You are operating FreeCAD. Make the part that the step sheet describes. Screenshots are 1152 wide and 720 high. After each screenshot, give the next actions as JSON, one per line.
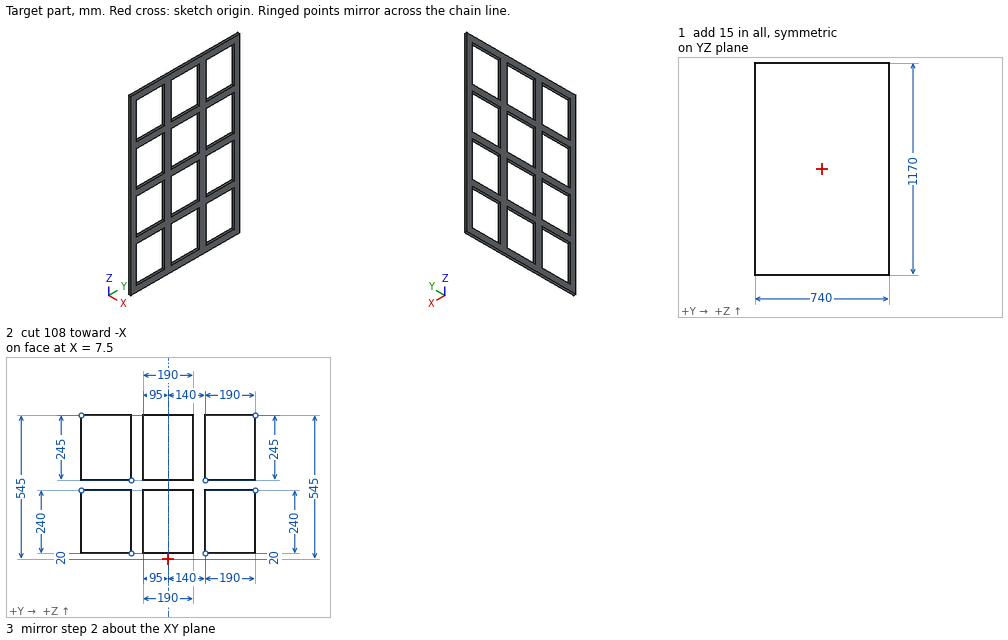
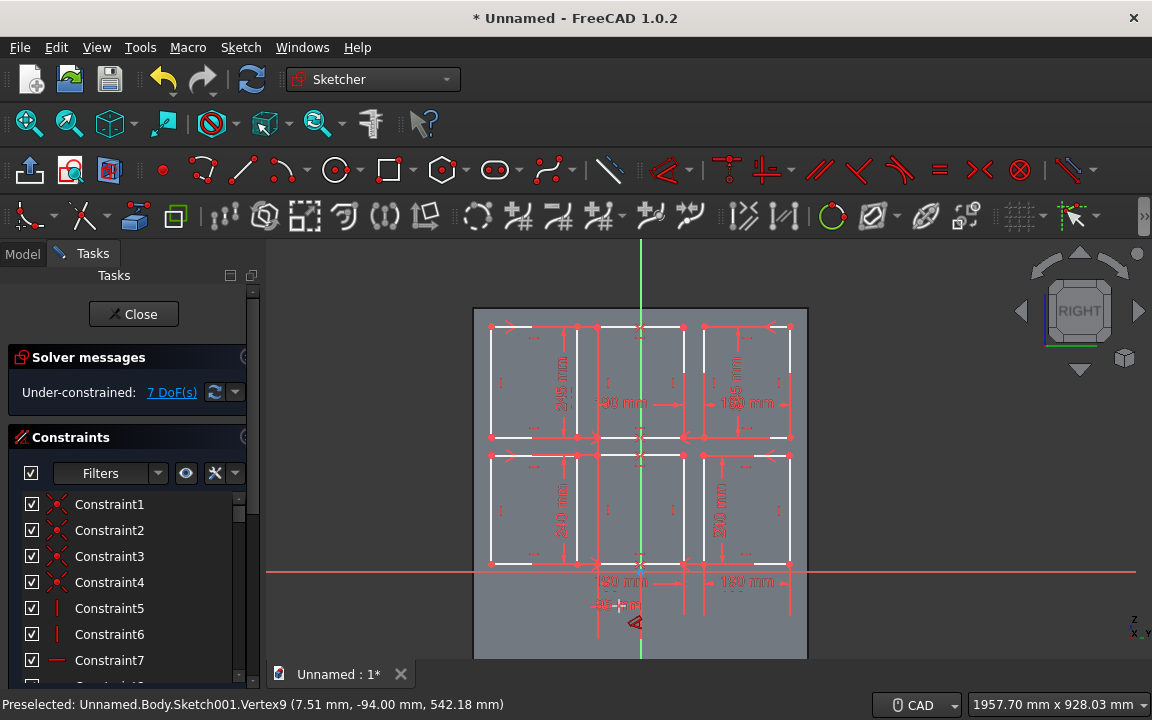
{"action": "left_click", "coordinate": [598, 455]}
{"action": "left_click", "coordinate": [619, 630]}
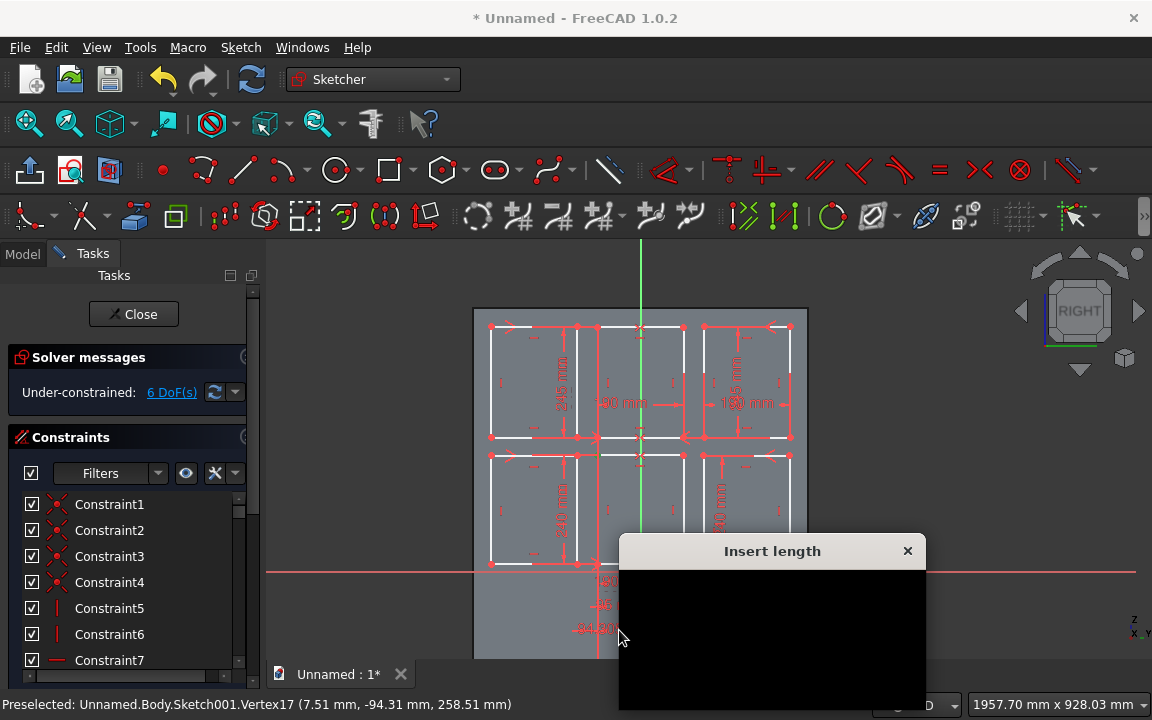
{"action": "type", "text": "95"}
{"action": "key", "text": "Return"}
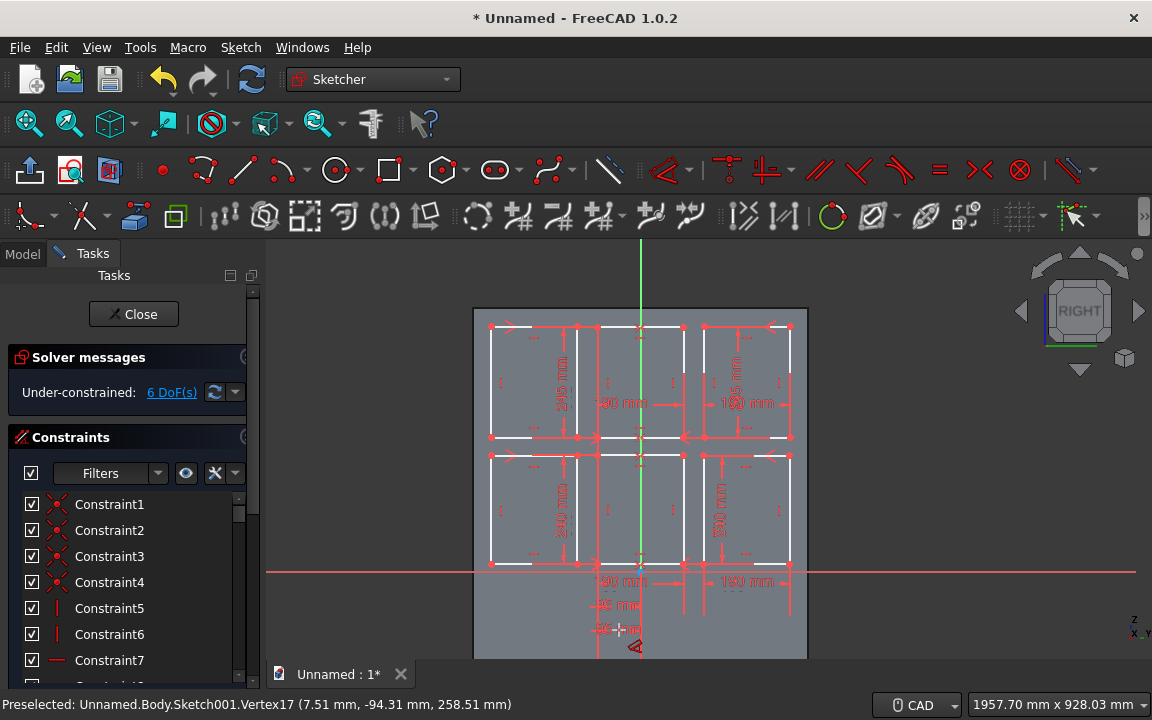
{"action": "scroll", "coordinate": [598, 564], "scroll_direction": "up", "scroll_amount": 8}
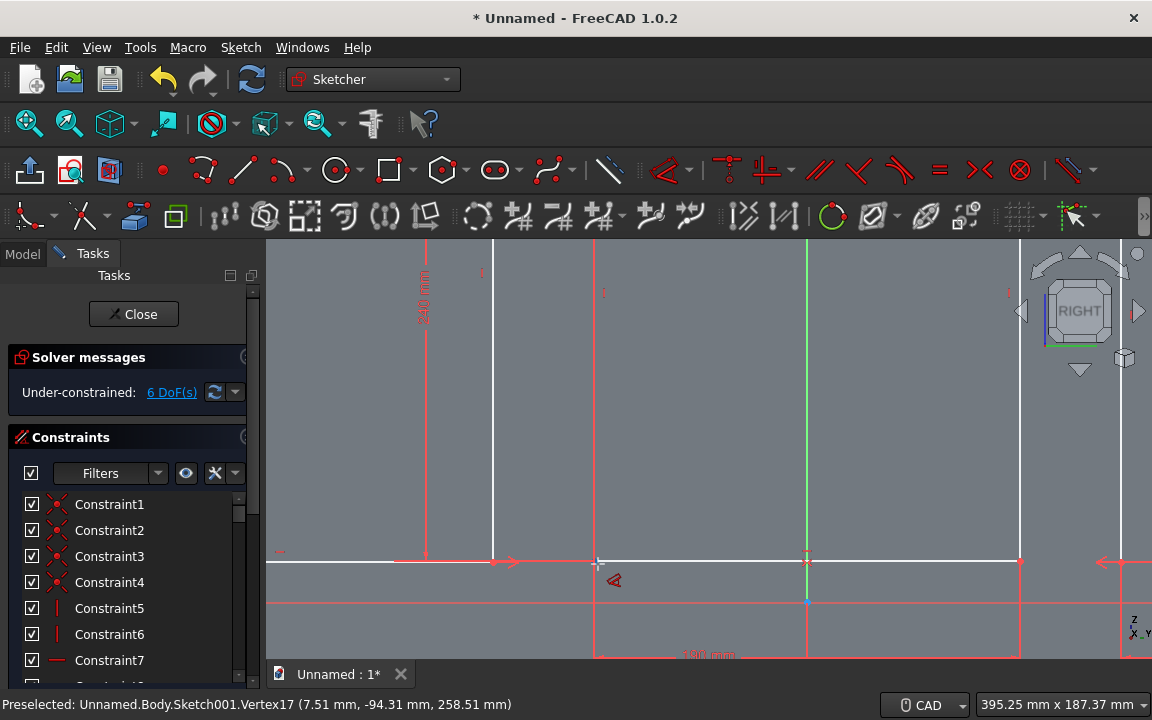
{"action": "left_click", "coordinate": [594, 561]}
{"action": "left_click", "coordinate": [560, 582]}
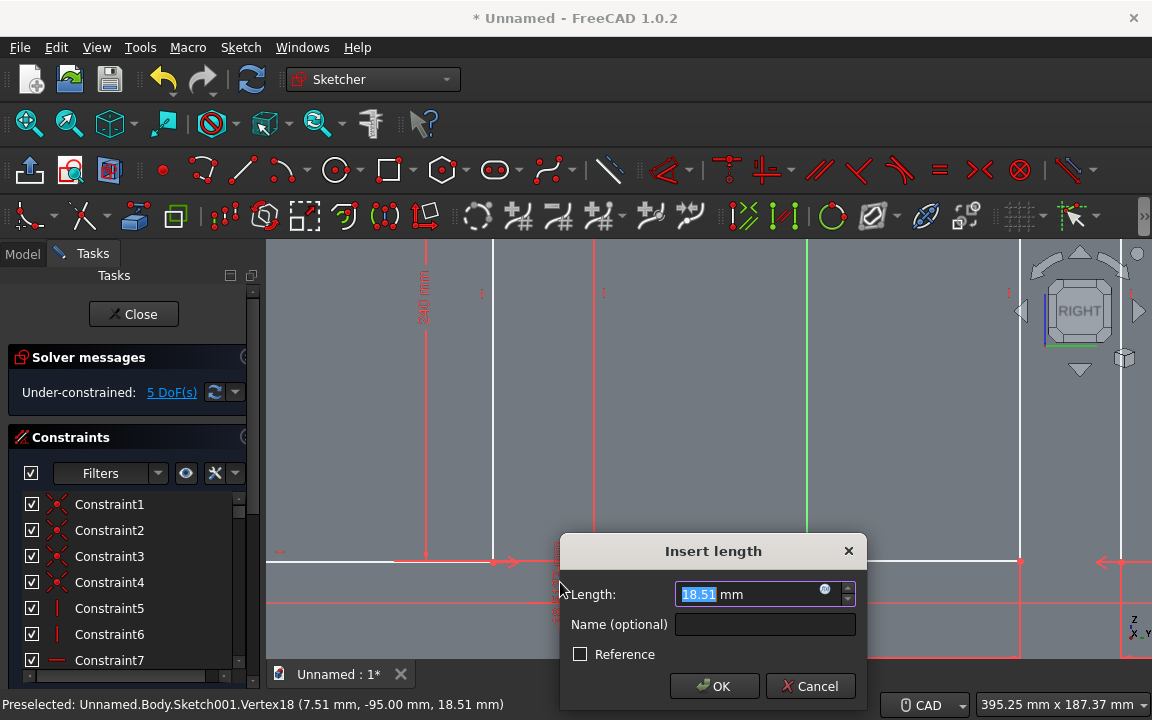
{"action": "type", "text": "20"}
{"action": "key", "text": "Return"}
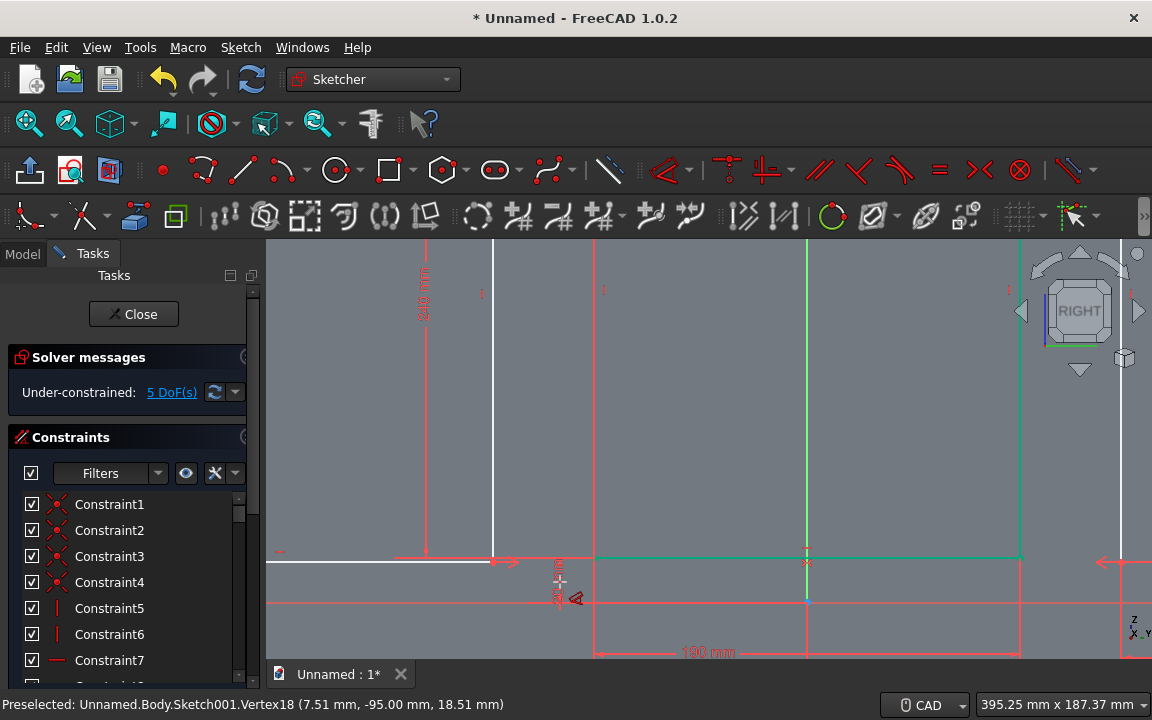
{"action": "scroll", "coordinate": [598, 565], "scroll_direction": "down", "scroll_amount": 8}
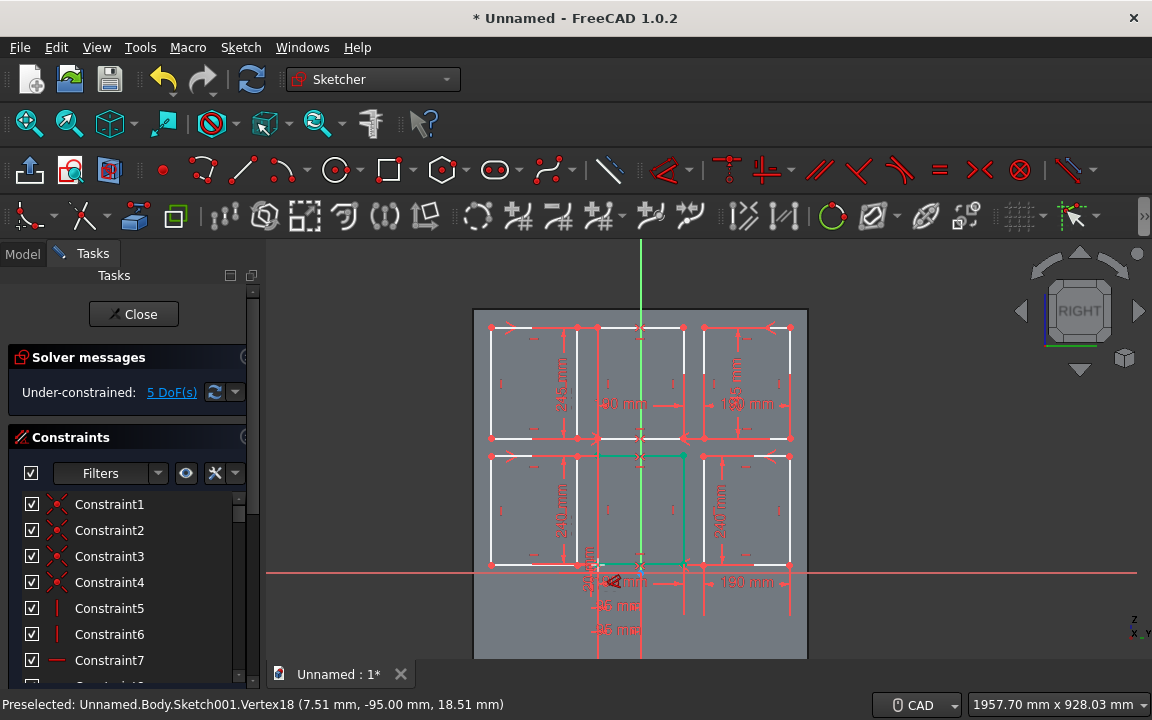
{"action": "scroll", "coordinate": [704, 565], "scroll_direction": "up", "scroll_amount": 8}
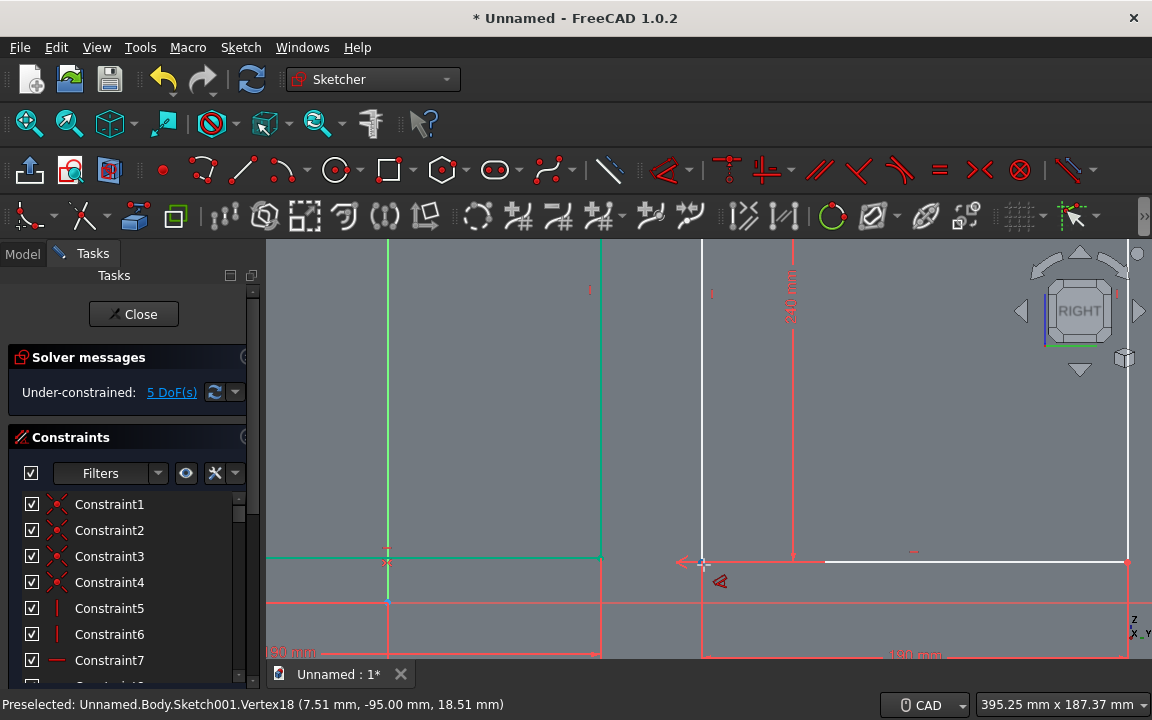
{"action": "left_click", "coordinate": [702, 562]}
{"action": "left_click", "coordinate": [736, 583]}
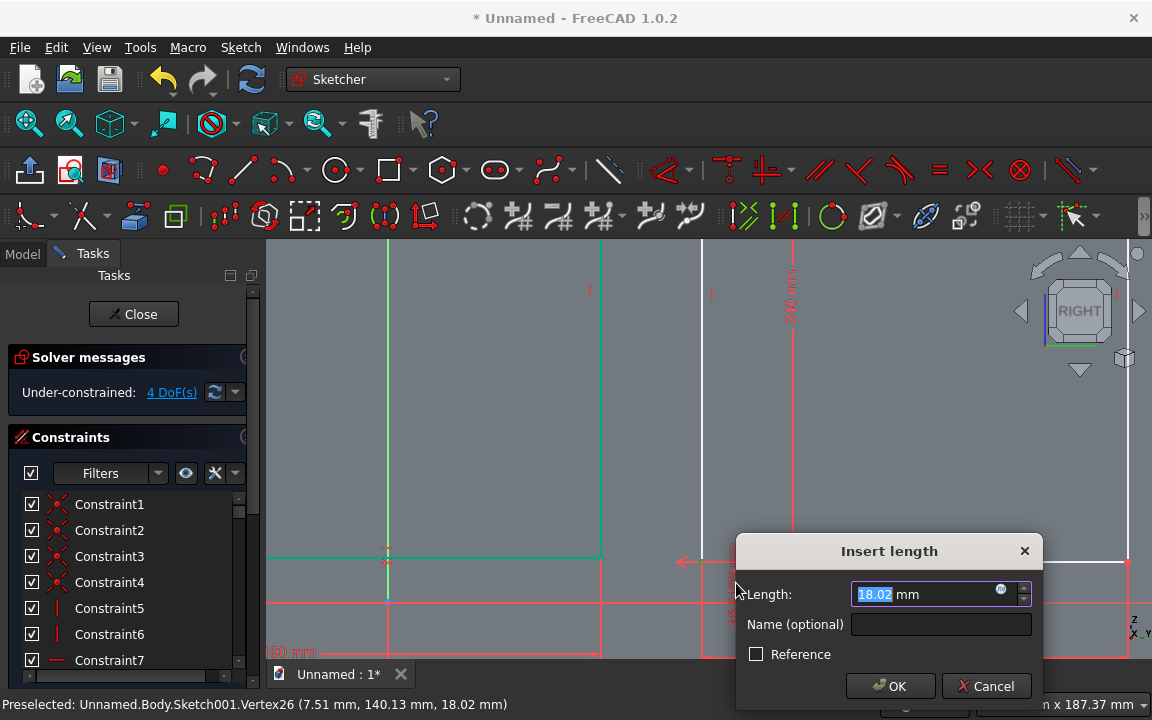
{"action": "type", "text": "20"}
{"action": "key", "text": "Return"}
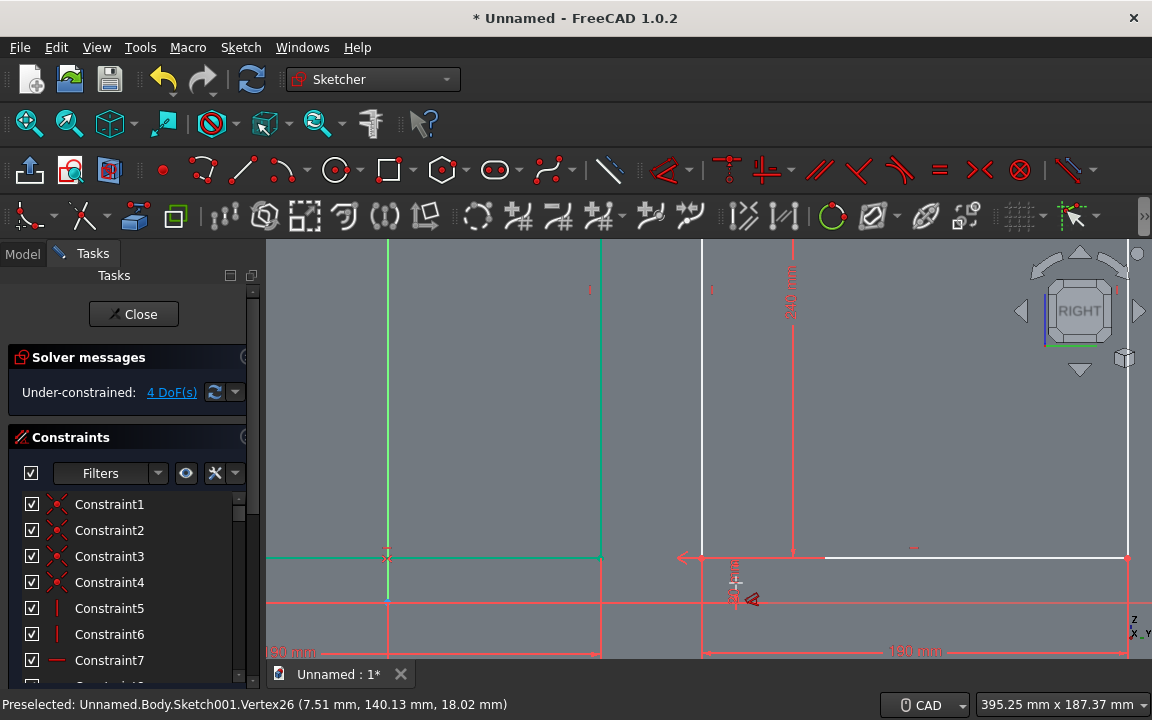
{"action": "scroll", "coordinate": [704, 565], "scroll_direction": "down", "scroll_amount": 8}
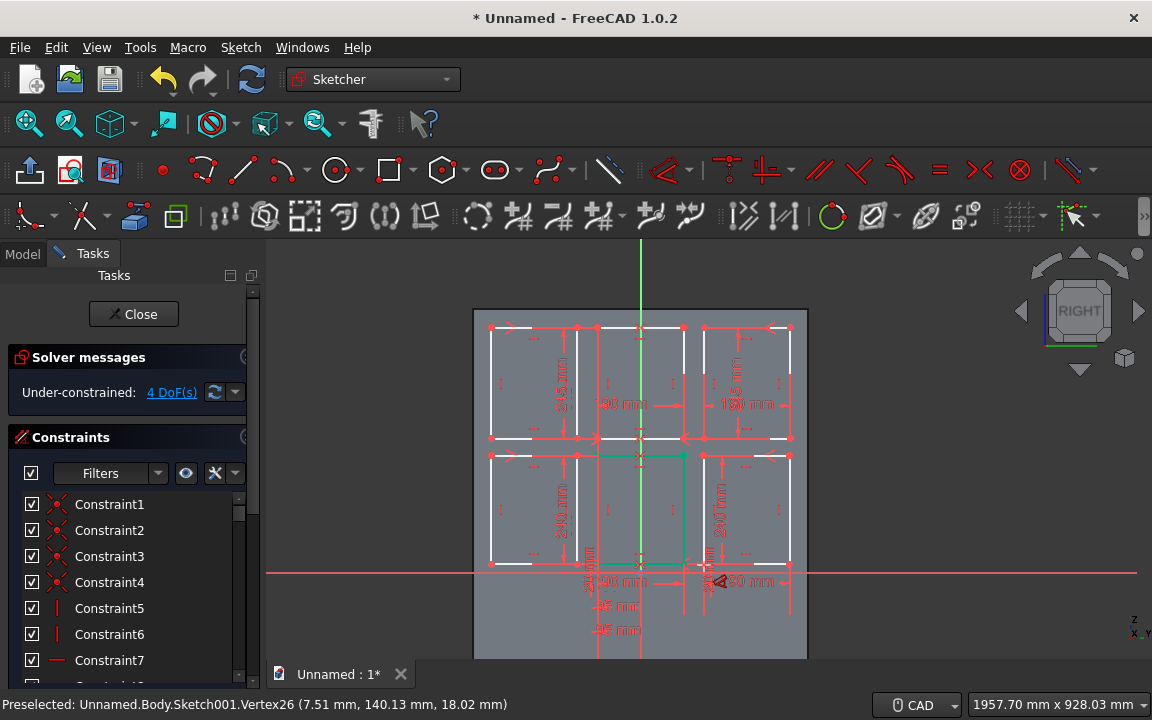
{"action": "left_click", "coordinate": [704, 328]}
{"action": "left_click", "coordinate": [695, 607]}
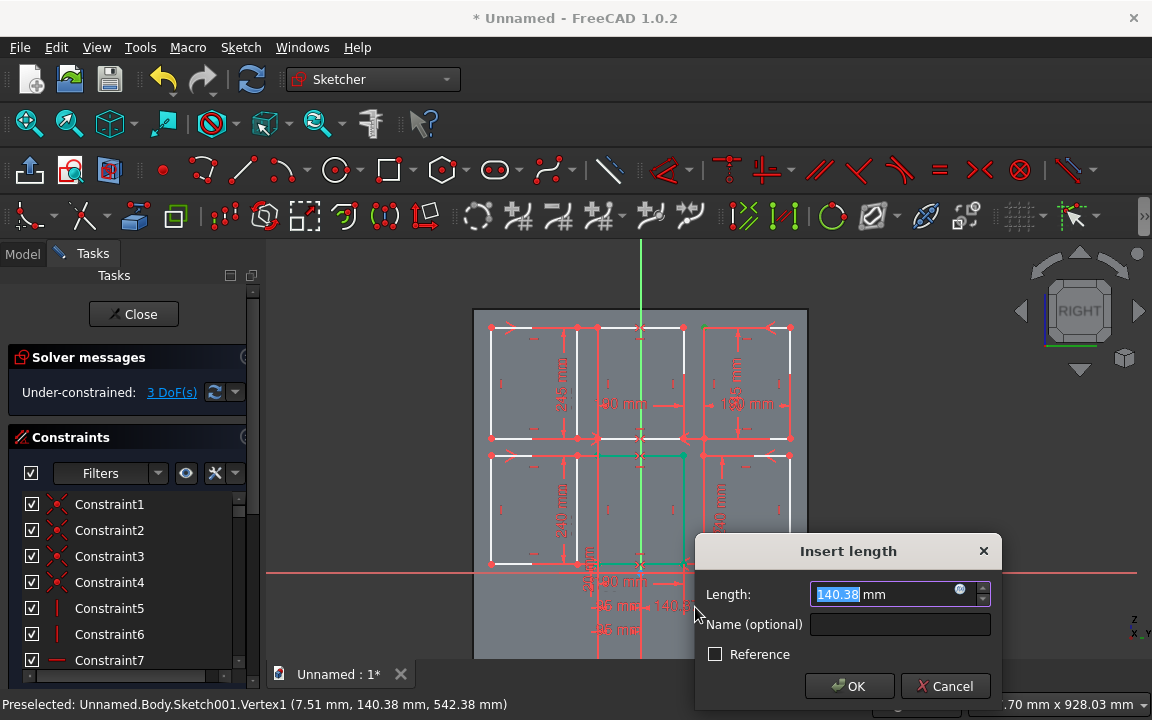
{"action": "type", "text": "140"}
{"action": "key", "text": "Return"}